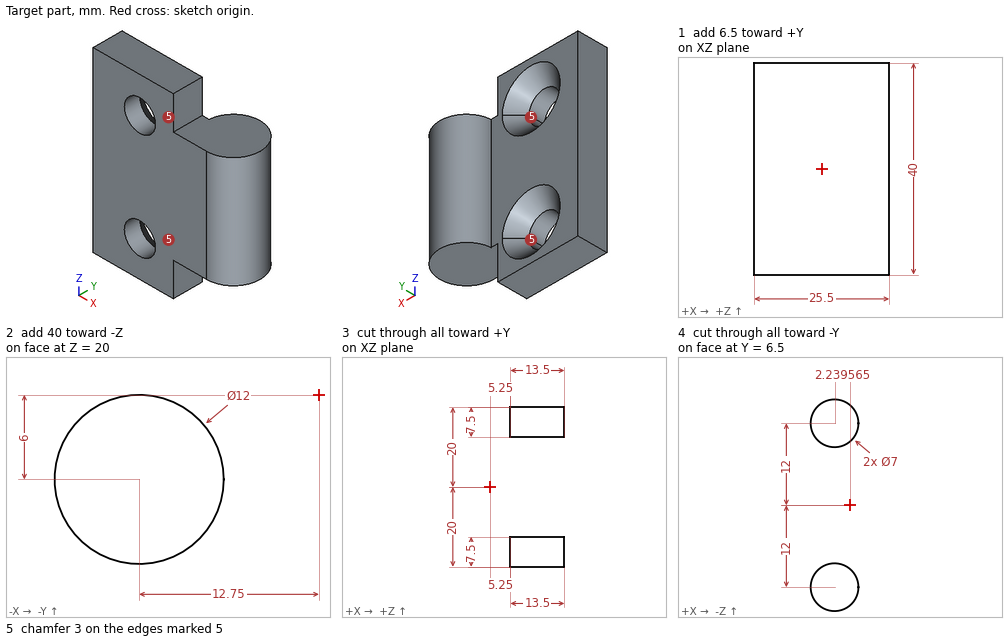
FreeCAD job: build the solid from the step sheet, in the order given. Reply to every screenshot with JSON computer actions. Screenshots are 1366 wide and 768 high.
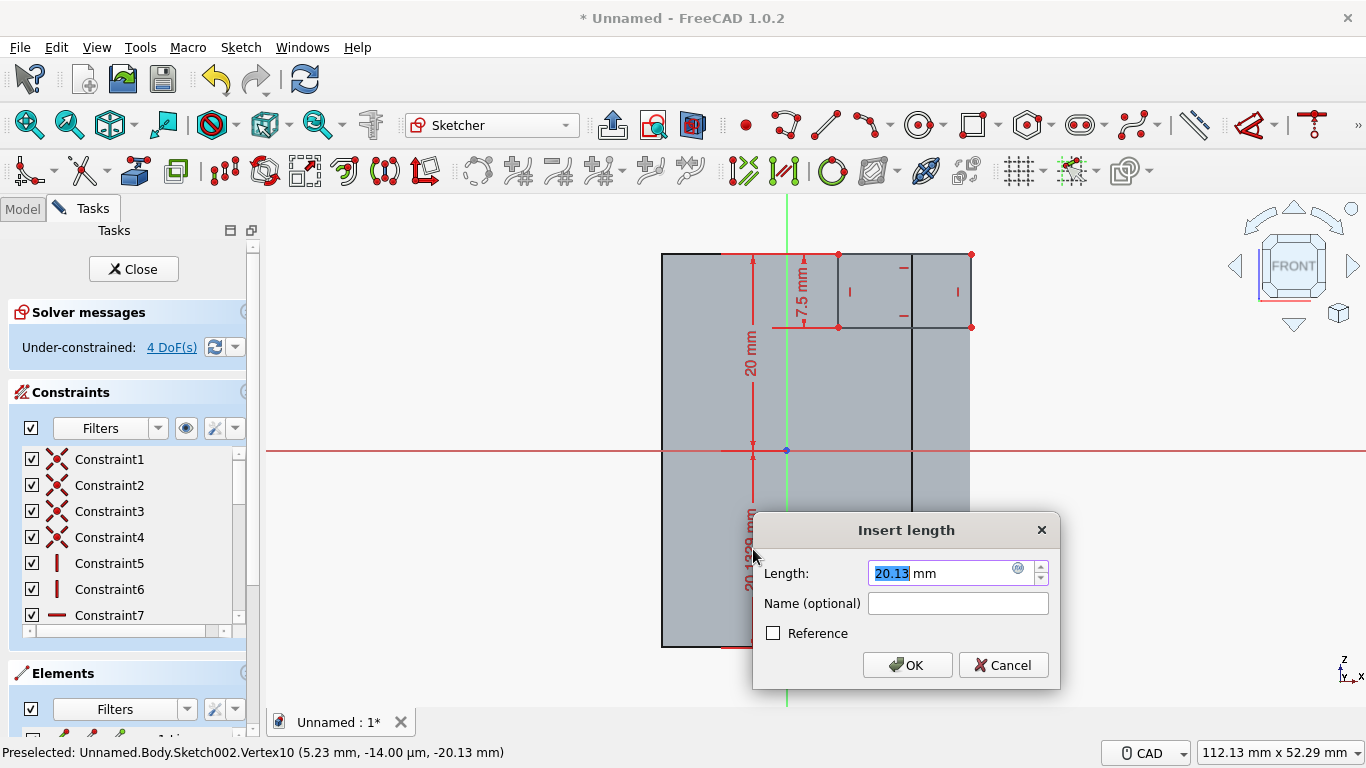
{"action": "type", "text": "20"}
{"action": "key", "text": "Return"}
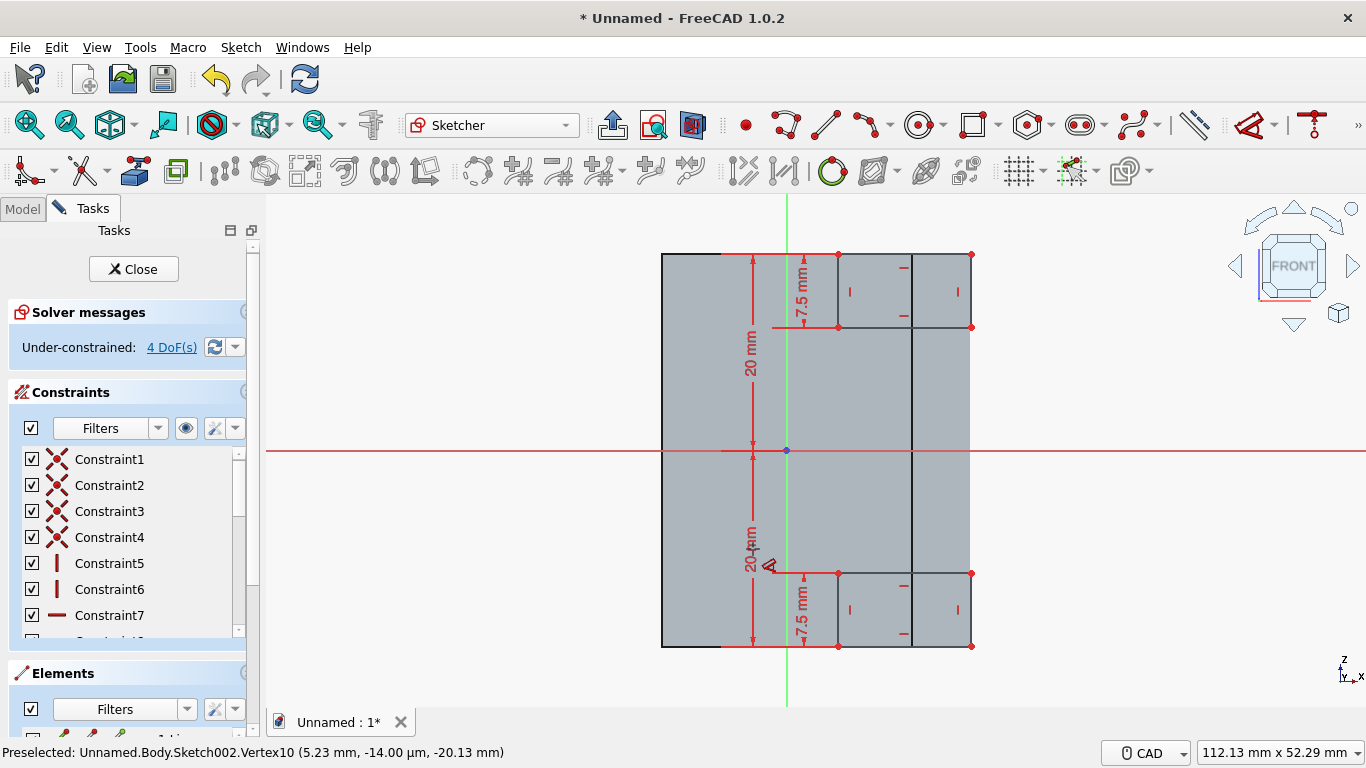
{"action": "left_click", "coordinate": [878, 328]}
{"action": "left_click", "coordinate": [904, 294]}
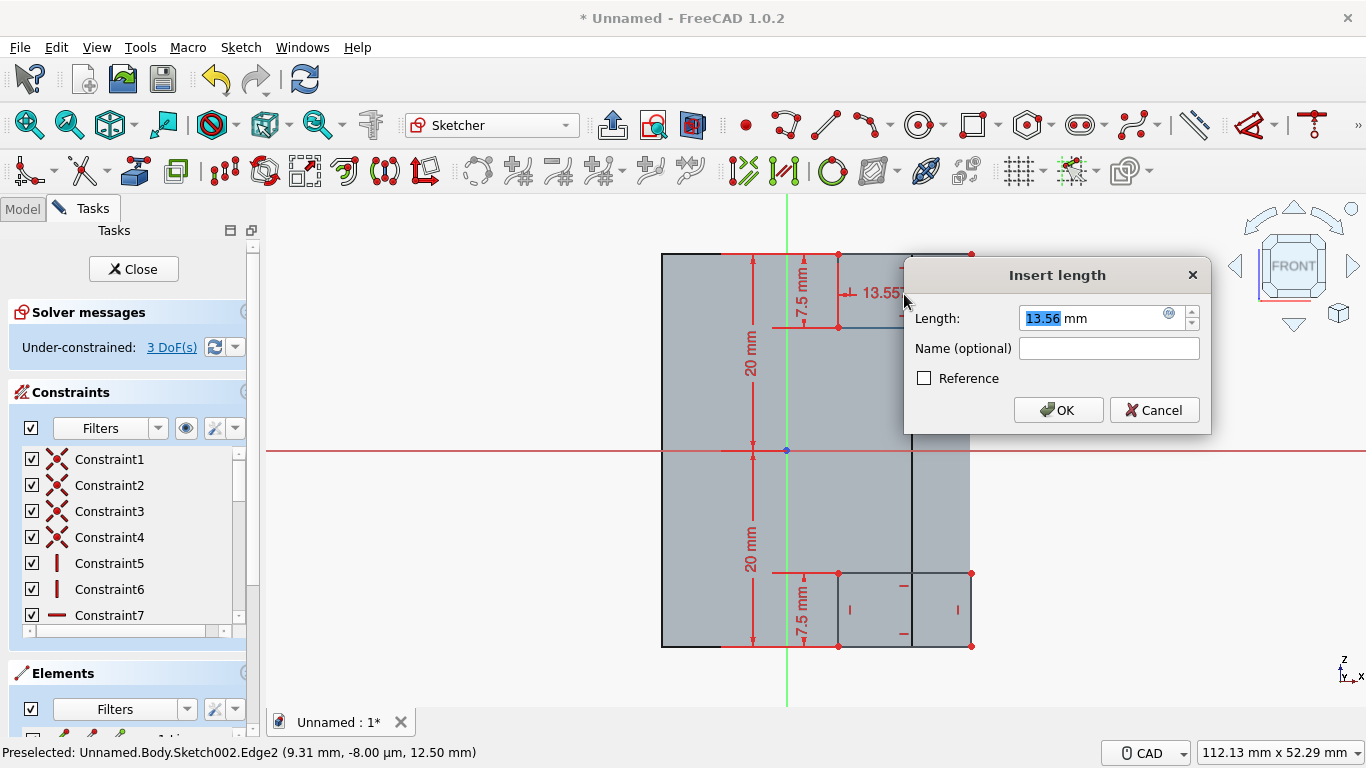
{"action": "type", "text": "13.5"}
{"action": "key", "text": "Return"}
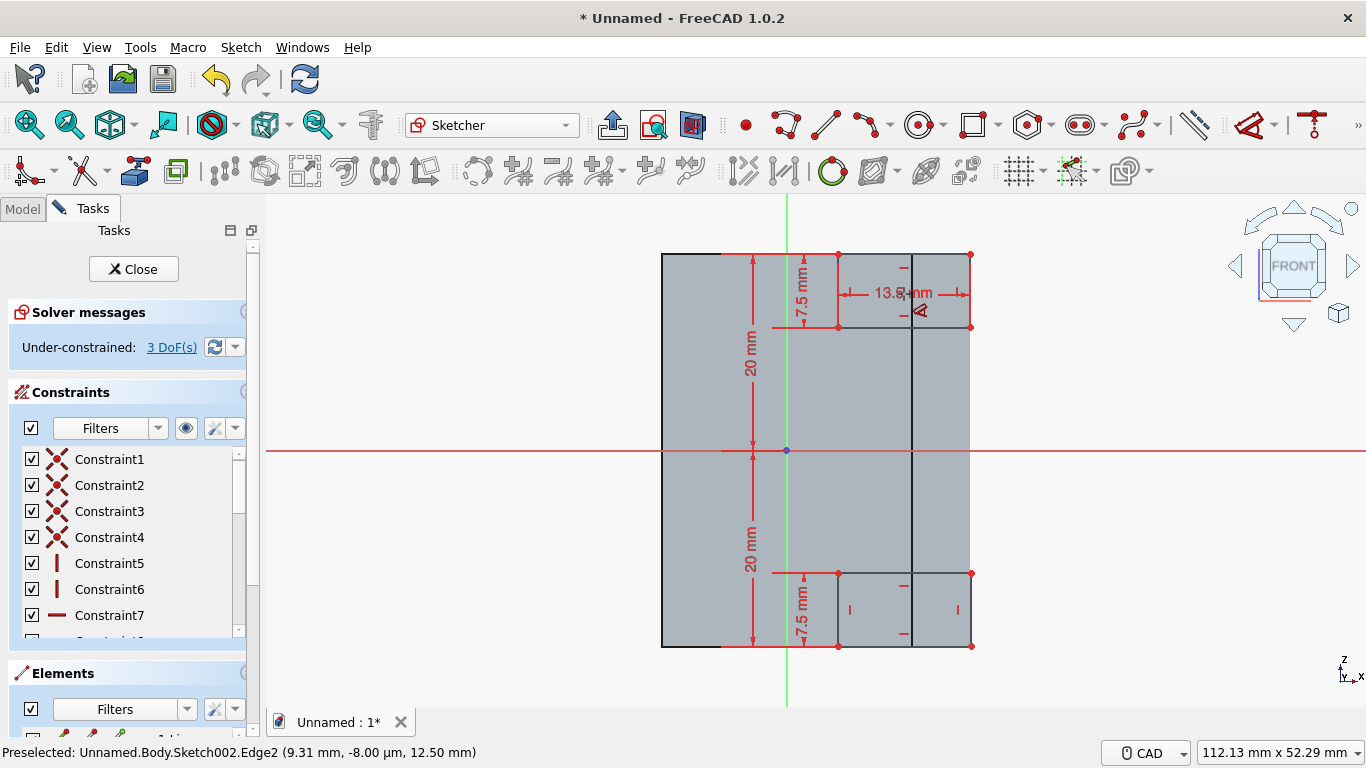
{"action": "left_click", "coordinate": [878, 647]}
{"action": "left_click", "coordinate": [904, 613]}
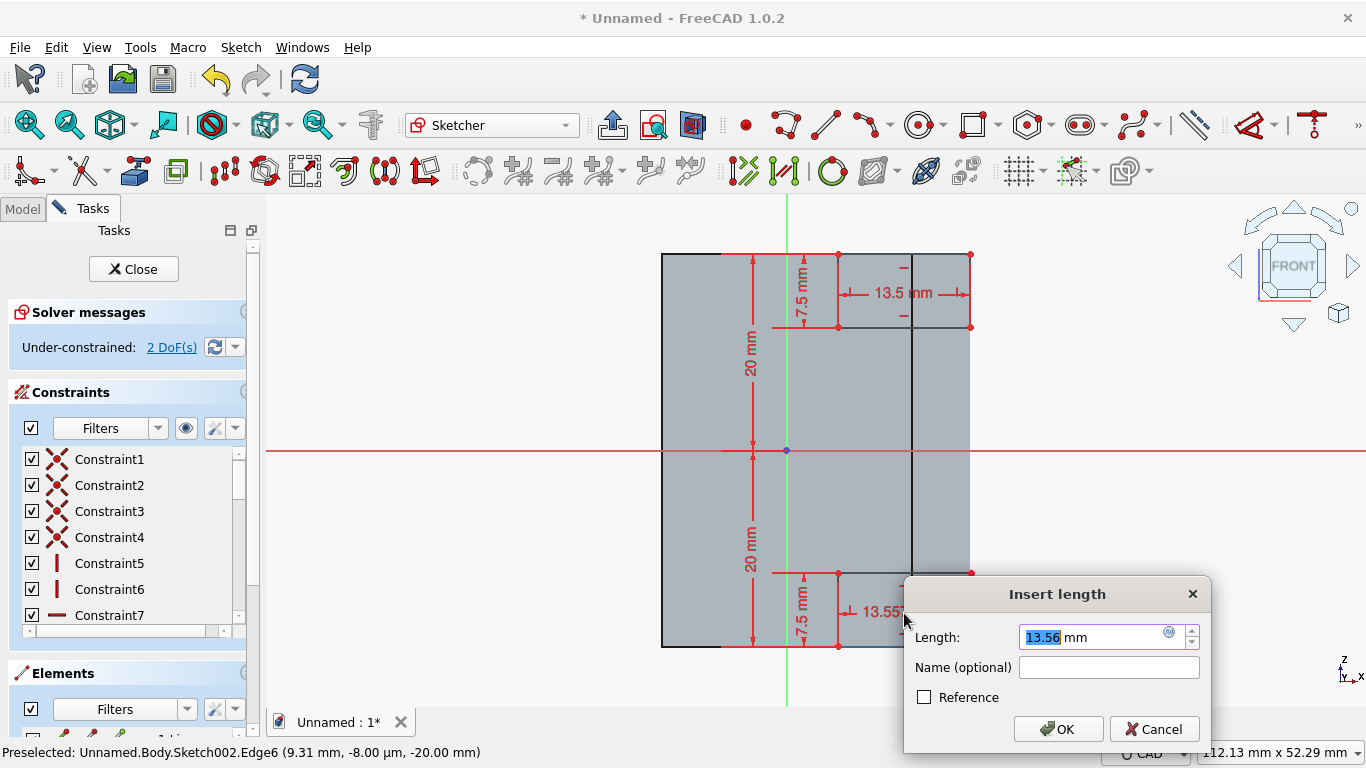
{"action": "type", "text": "13.5"}
{"action": "key", "text": "Return"}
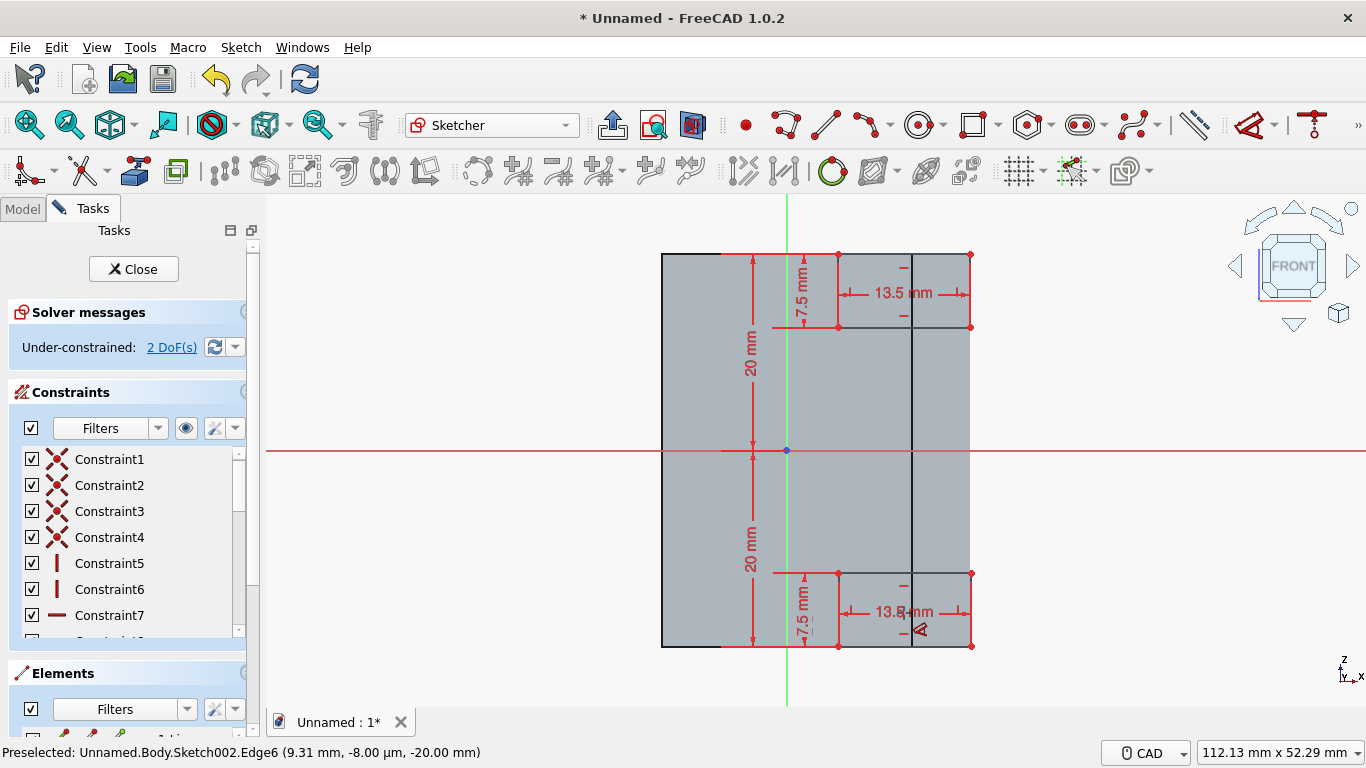
{"action": "left_click", "coordinate": [838, 254]}
{"action": "left_click", "coordinate": [812, 485]}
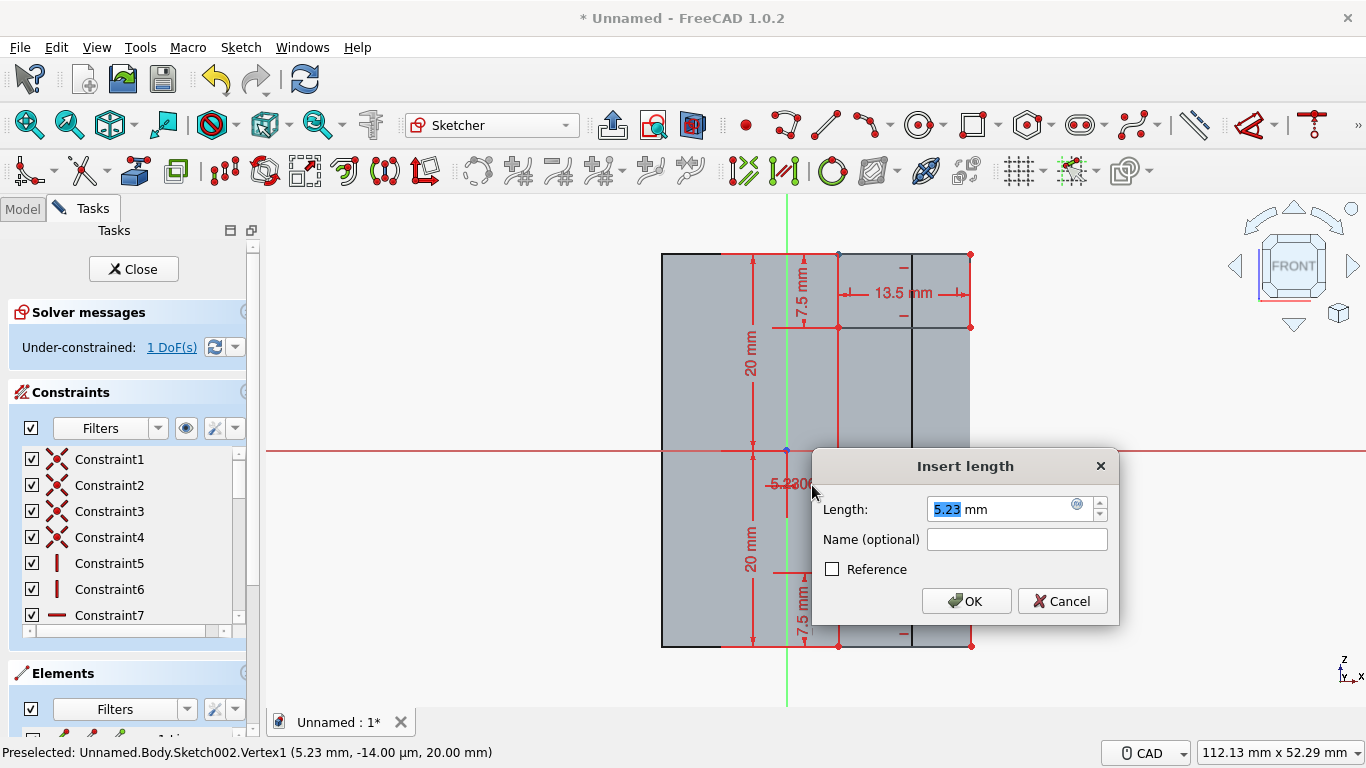
{"action": "type", "text": "5.25"}
{"action": "key", "text": "Return"}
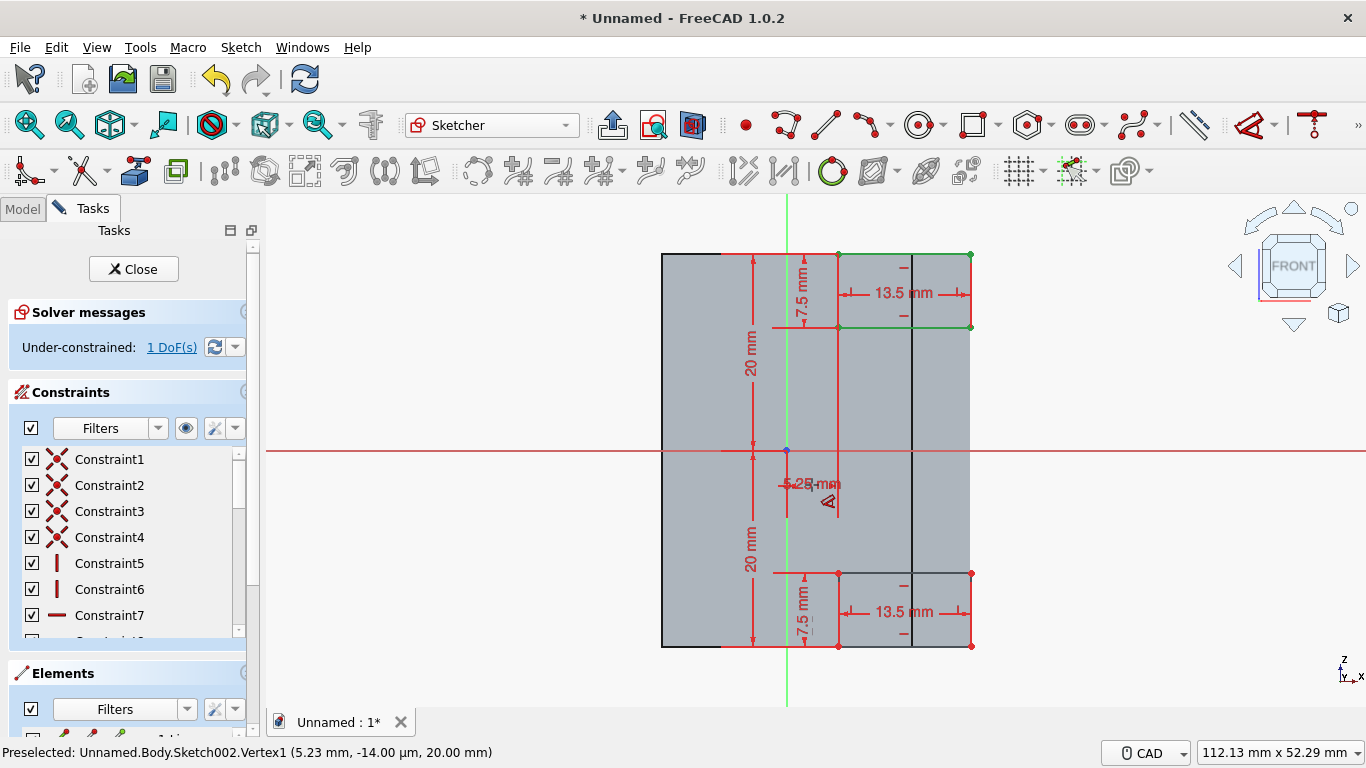
{"action": "left_click", "coordinate": [839, 573]}
{"action": "left_click", "coordinate": [813, 417]}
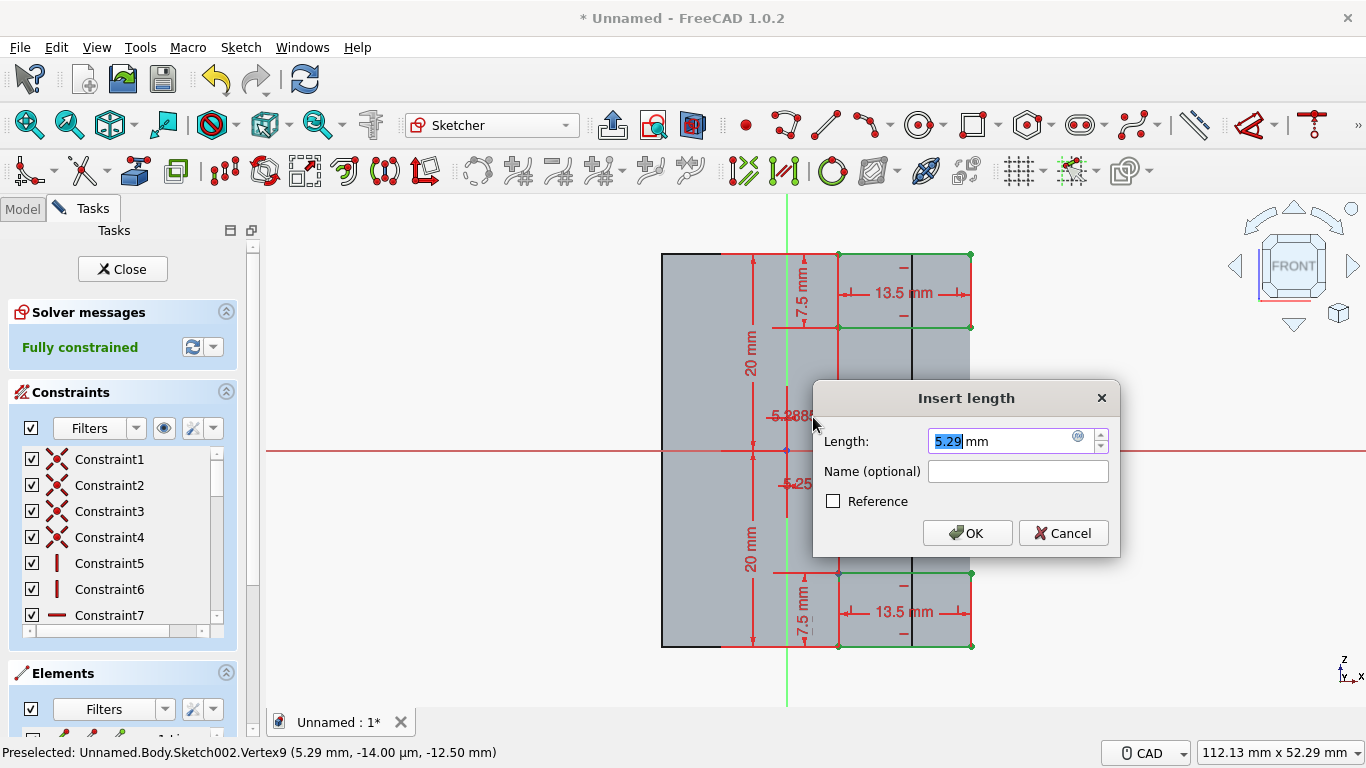
{"action": "type", "text": "5.25"}
{"action": "key", "text": "Return"}
{"action": "key", "text": "Escape"}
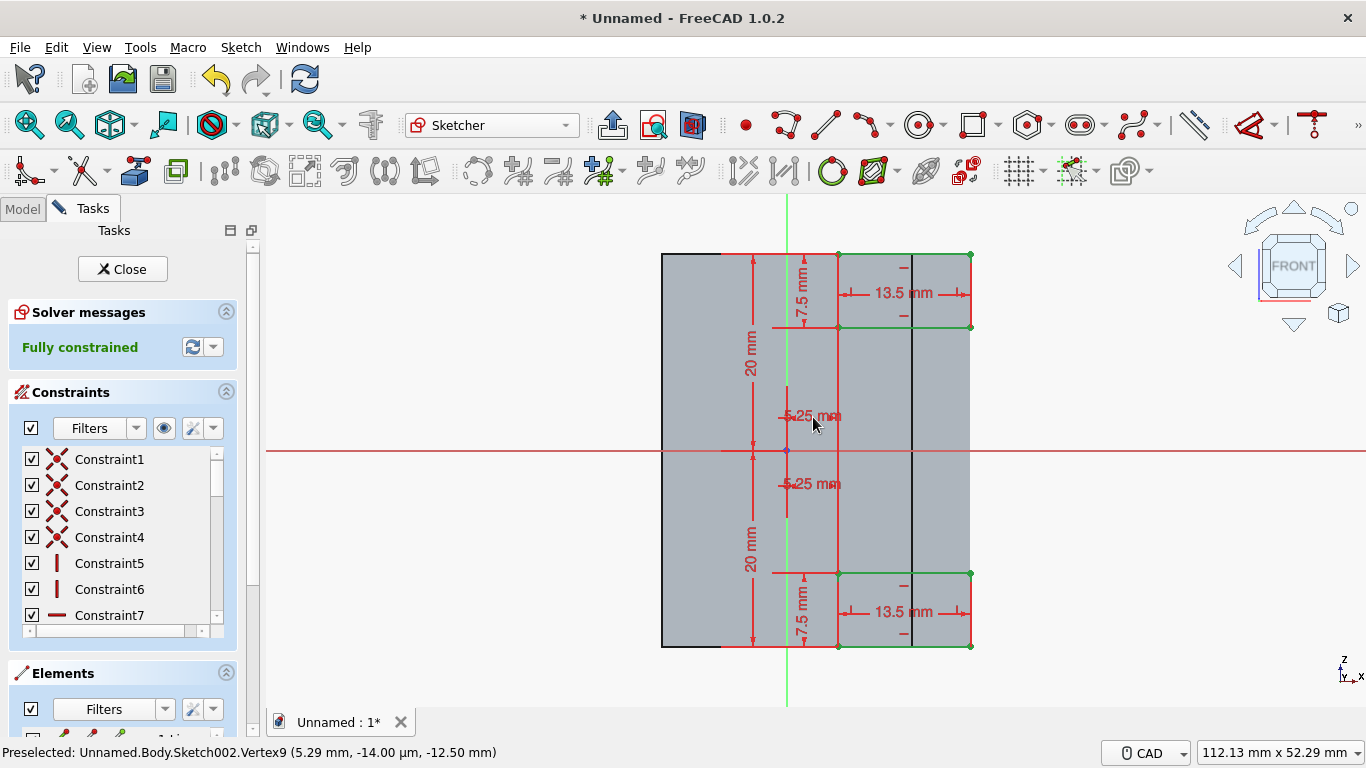
{"action": "left_click", "coordinate": [123, 269]}